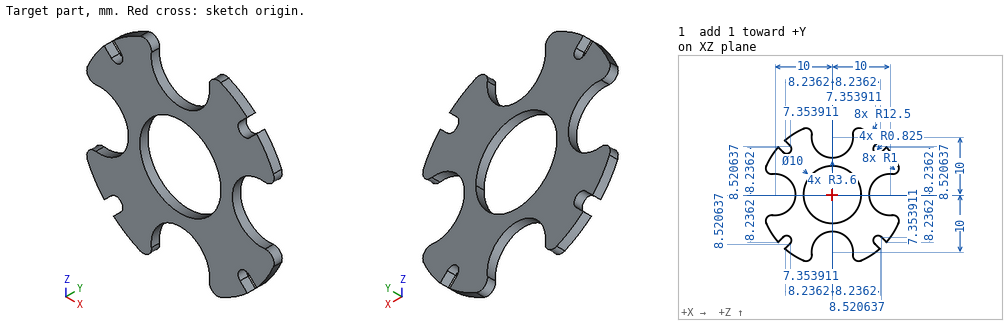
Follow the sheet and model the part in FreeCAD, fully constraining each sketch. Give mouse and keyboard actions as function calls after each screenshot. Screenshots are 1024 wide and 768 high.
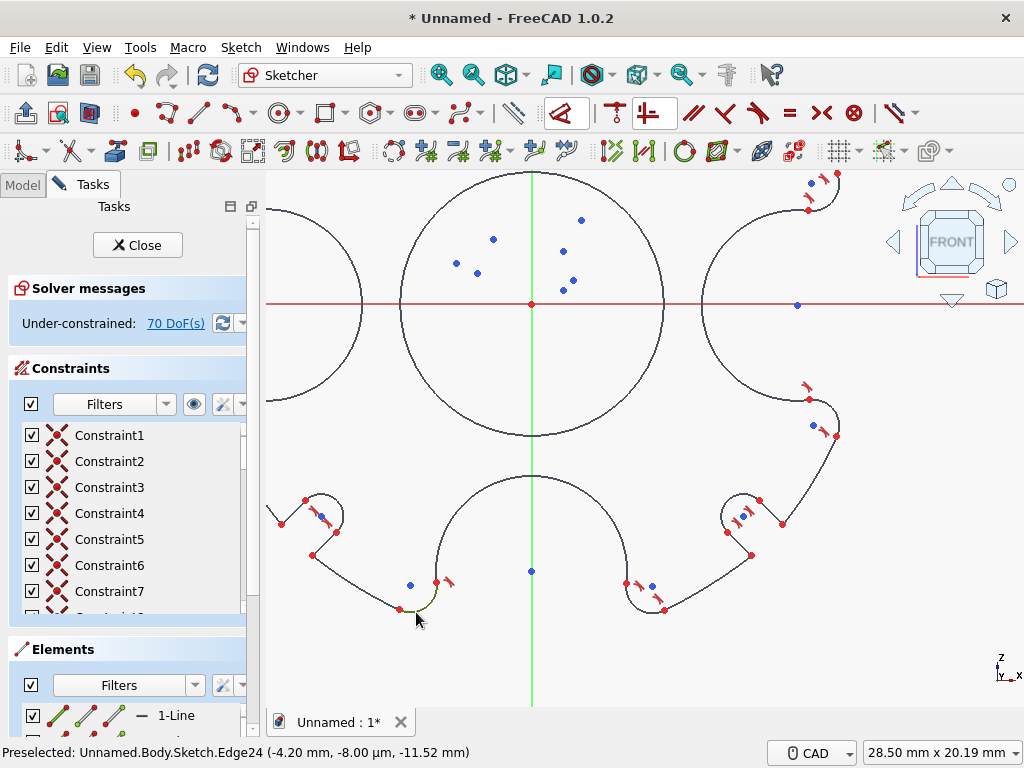
click(337, 574)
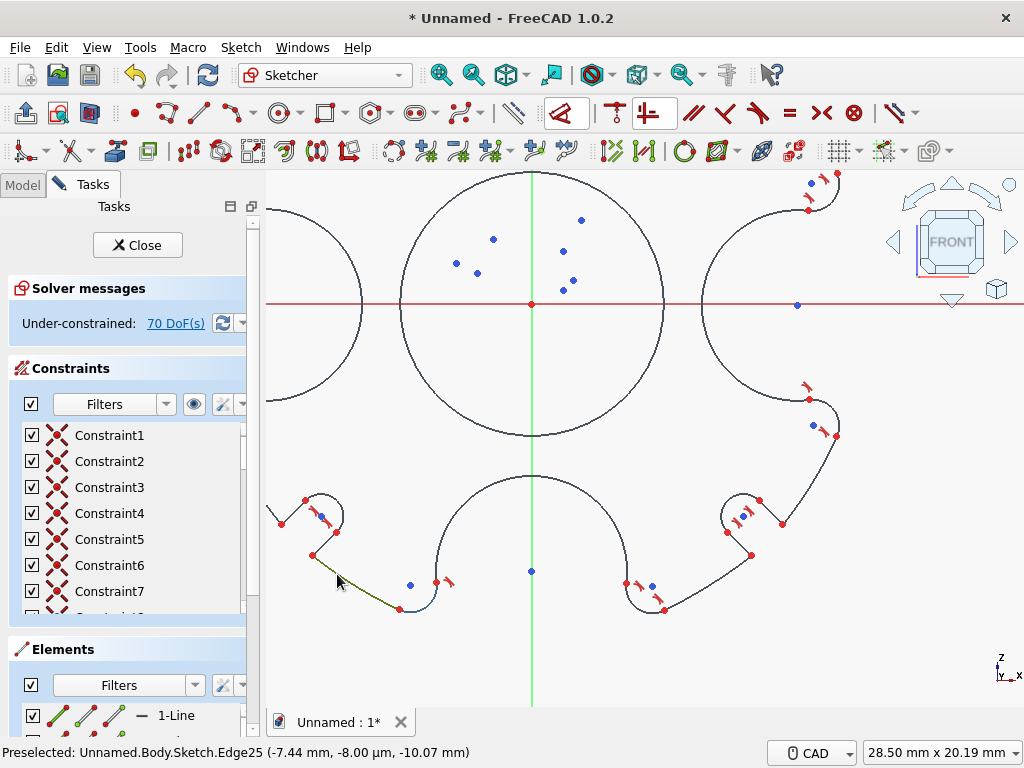
click(758, 114)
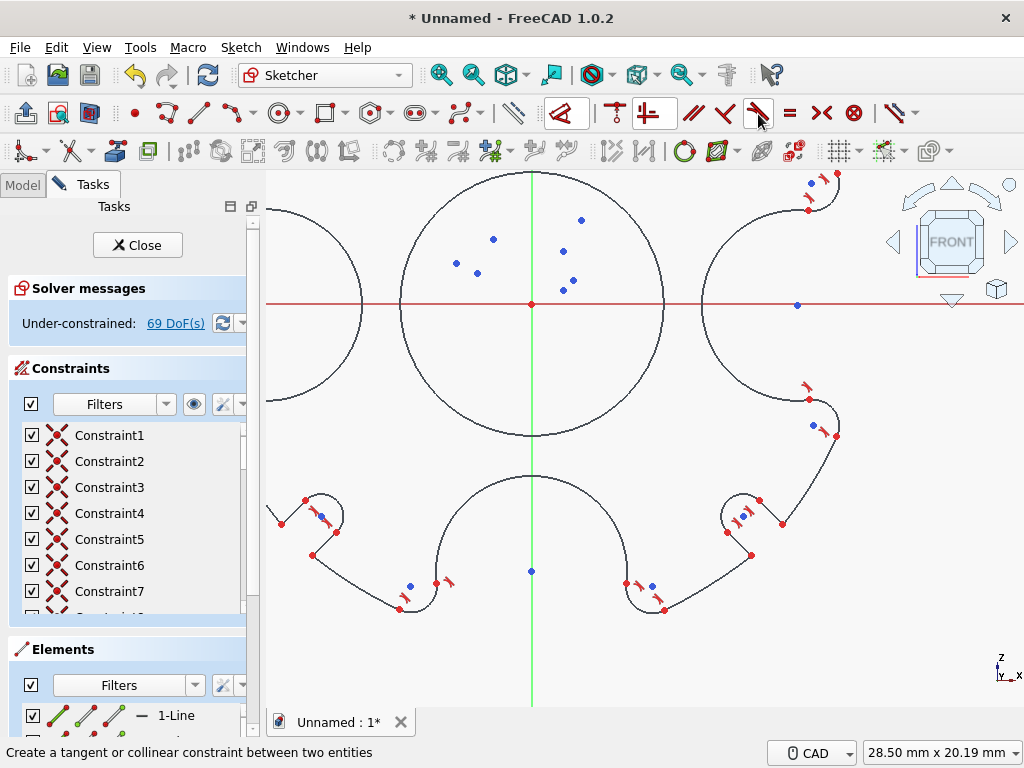
scroll(631, 602, down, 3)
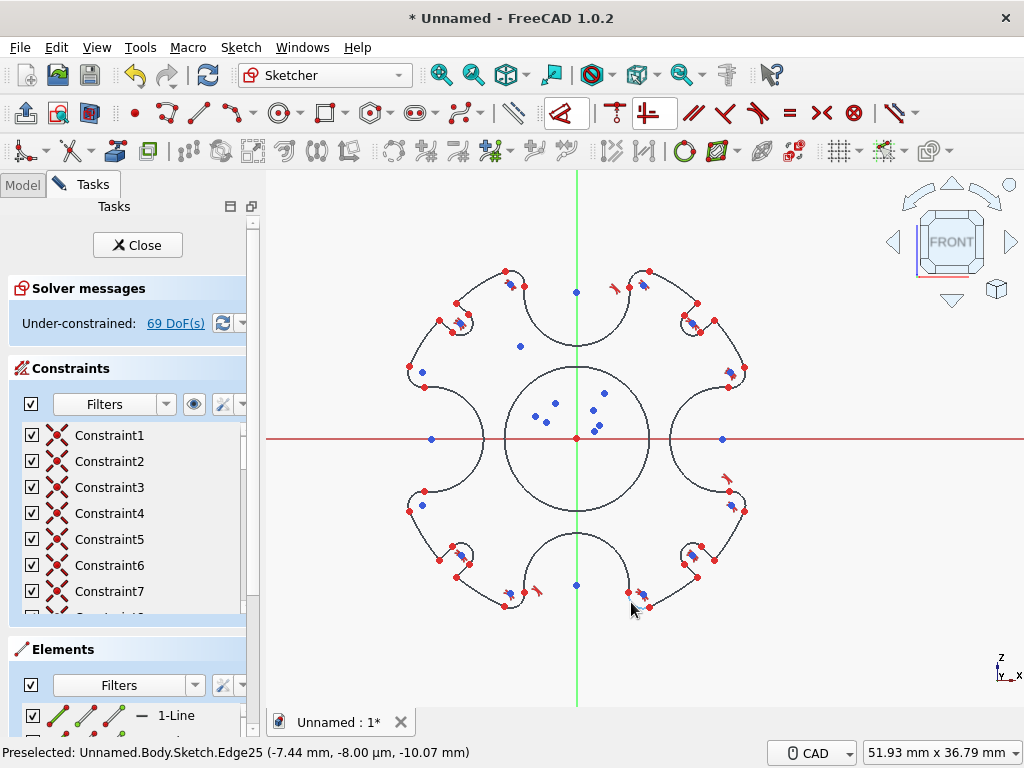
click(417, 527)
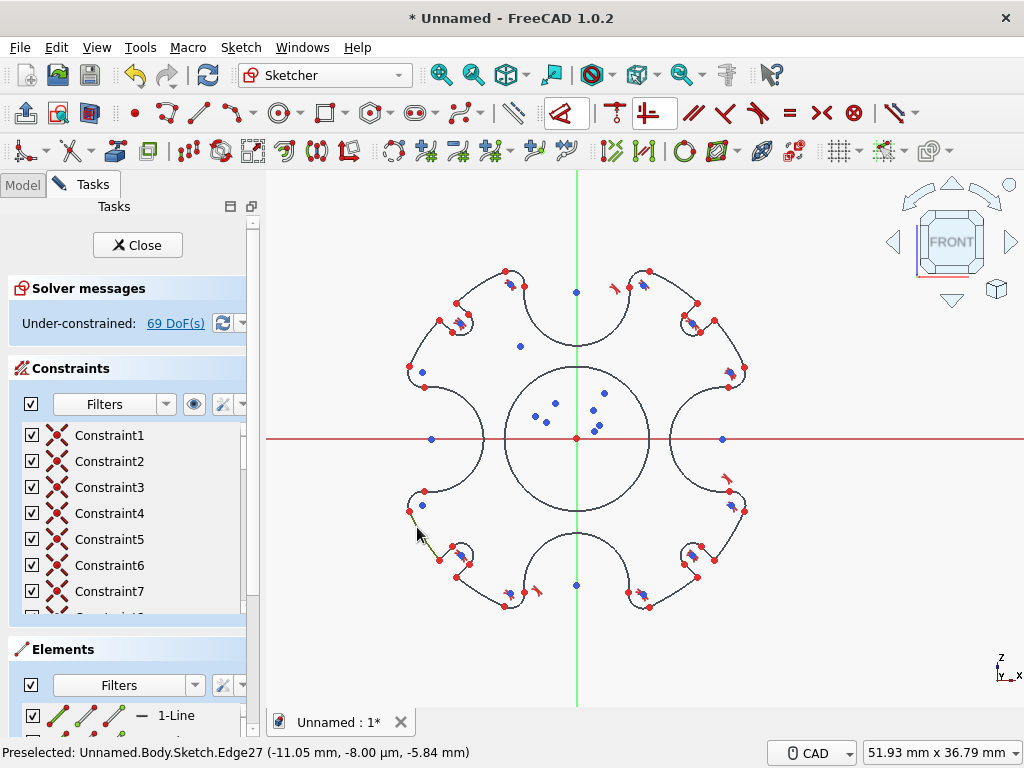
scroll(416, 493, up, 3)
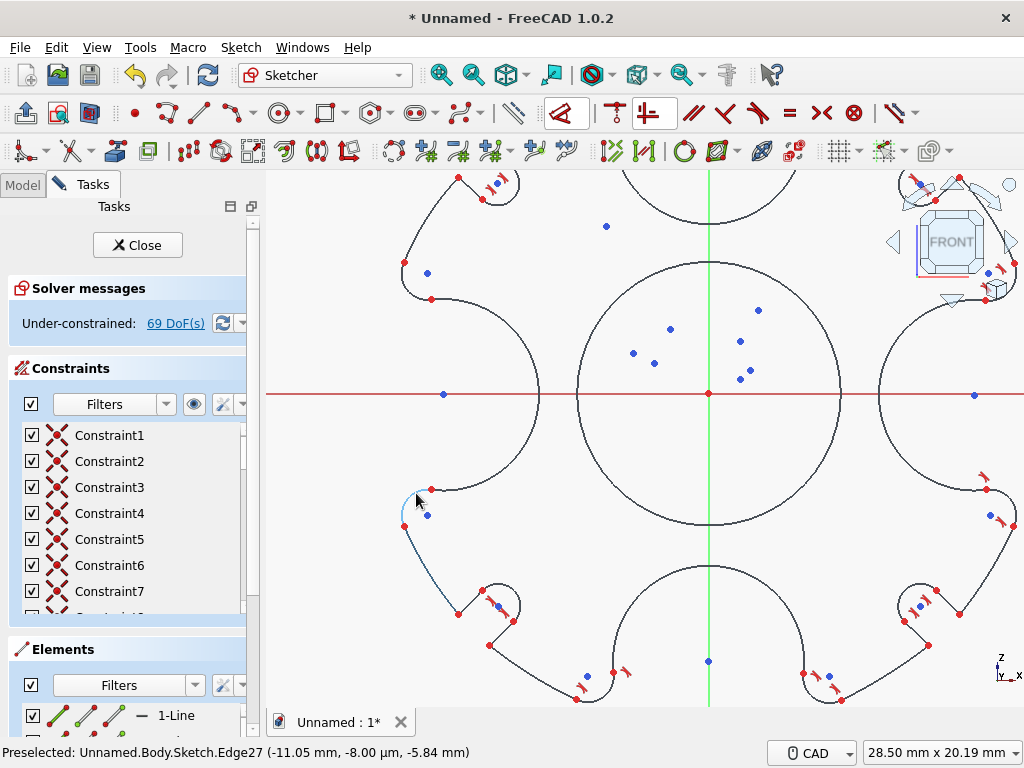
click(416, 493)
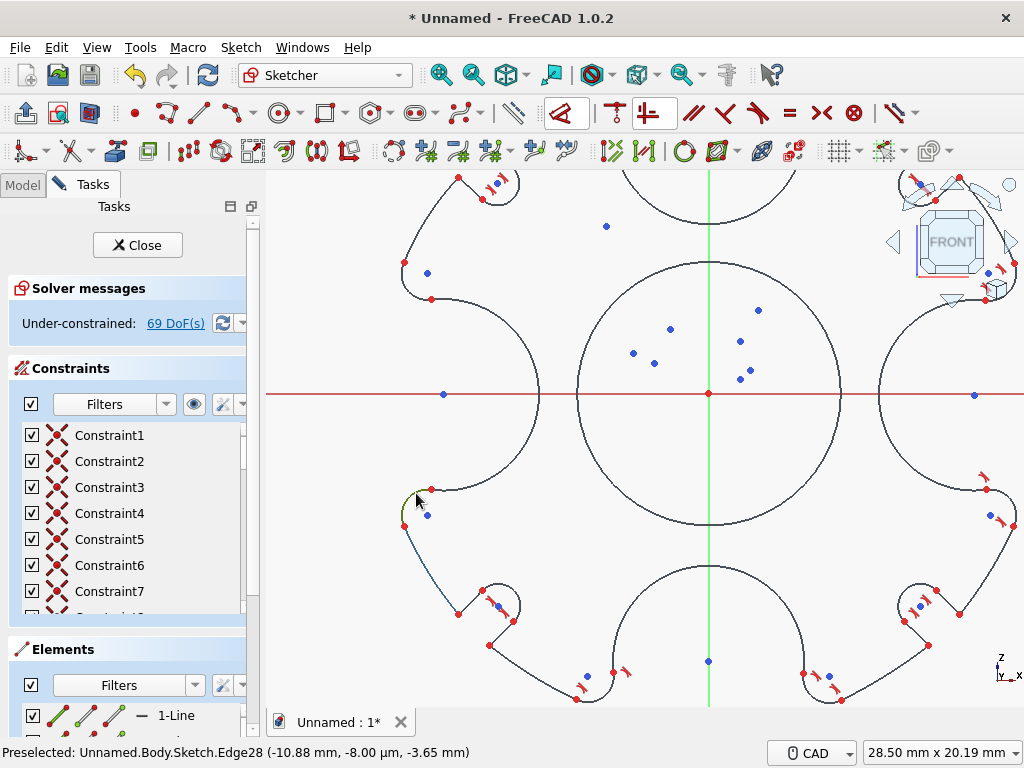
key(t)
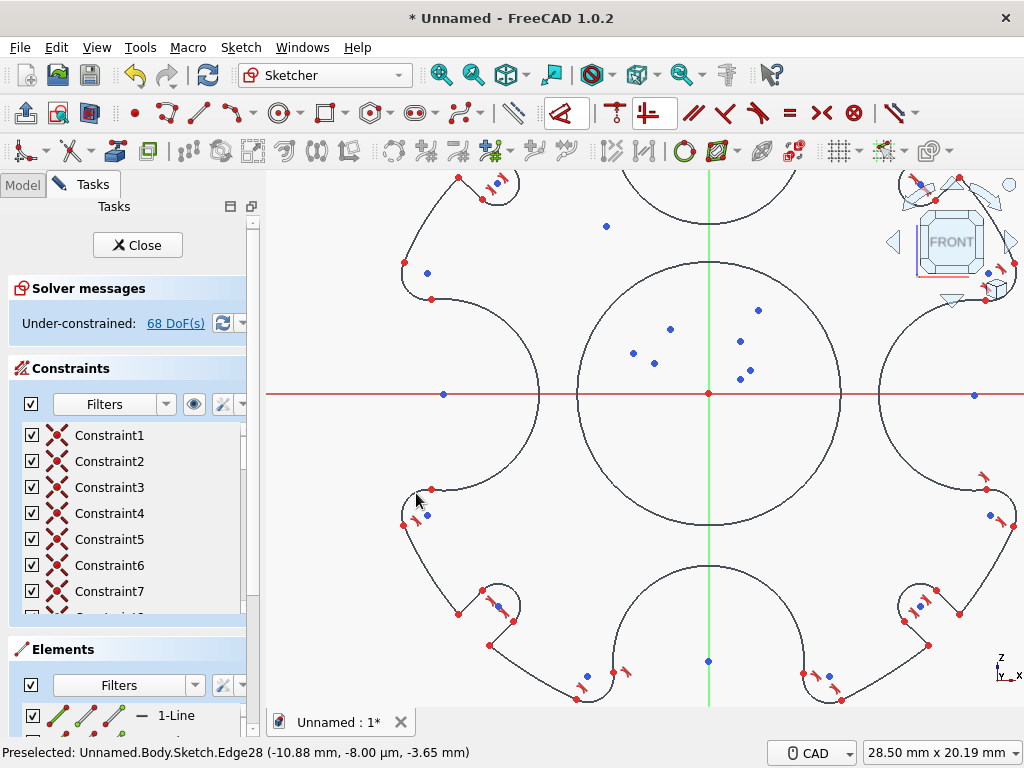
click(416, 492)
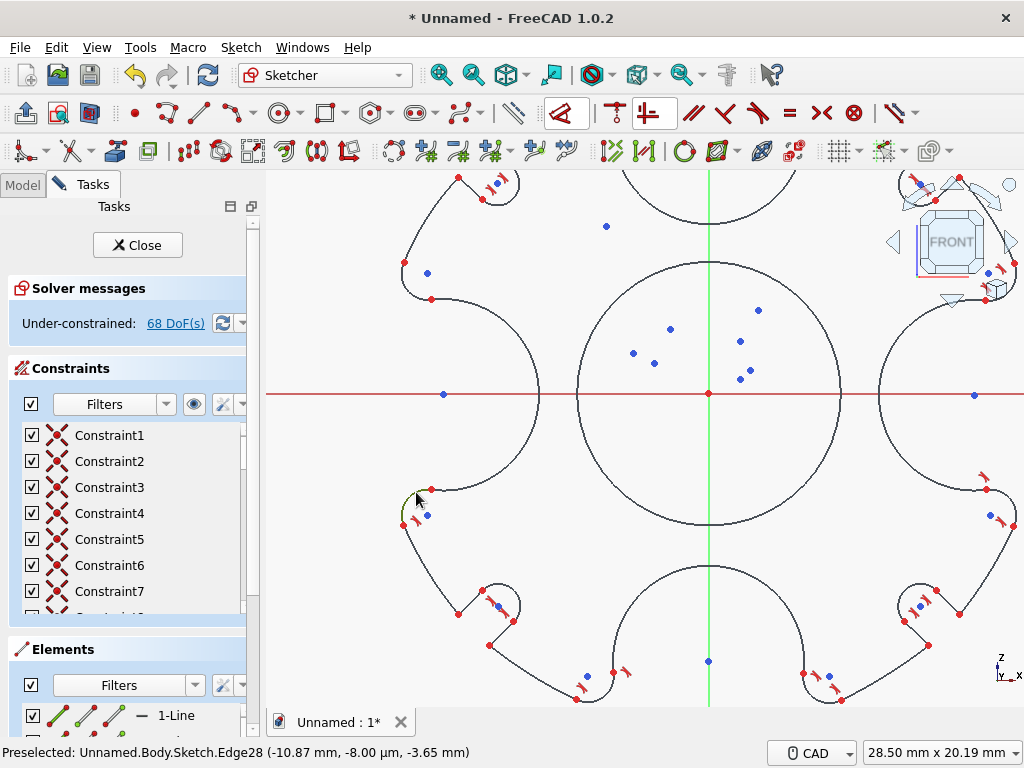
click(518, 455)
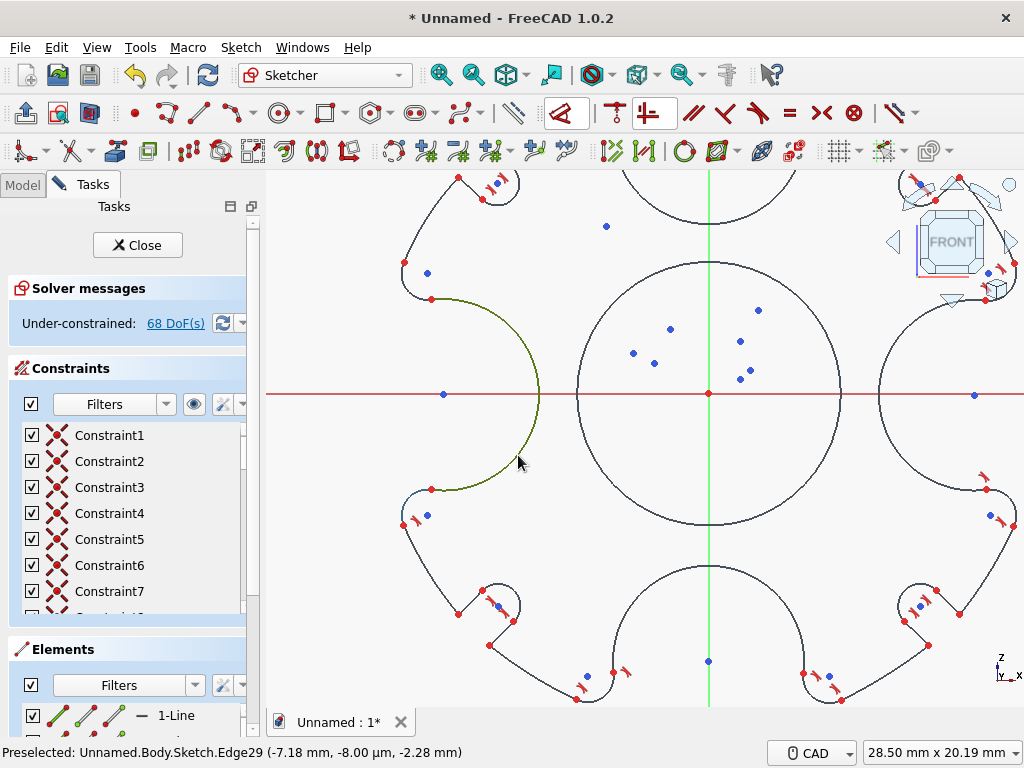
key(t)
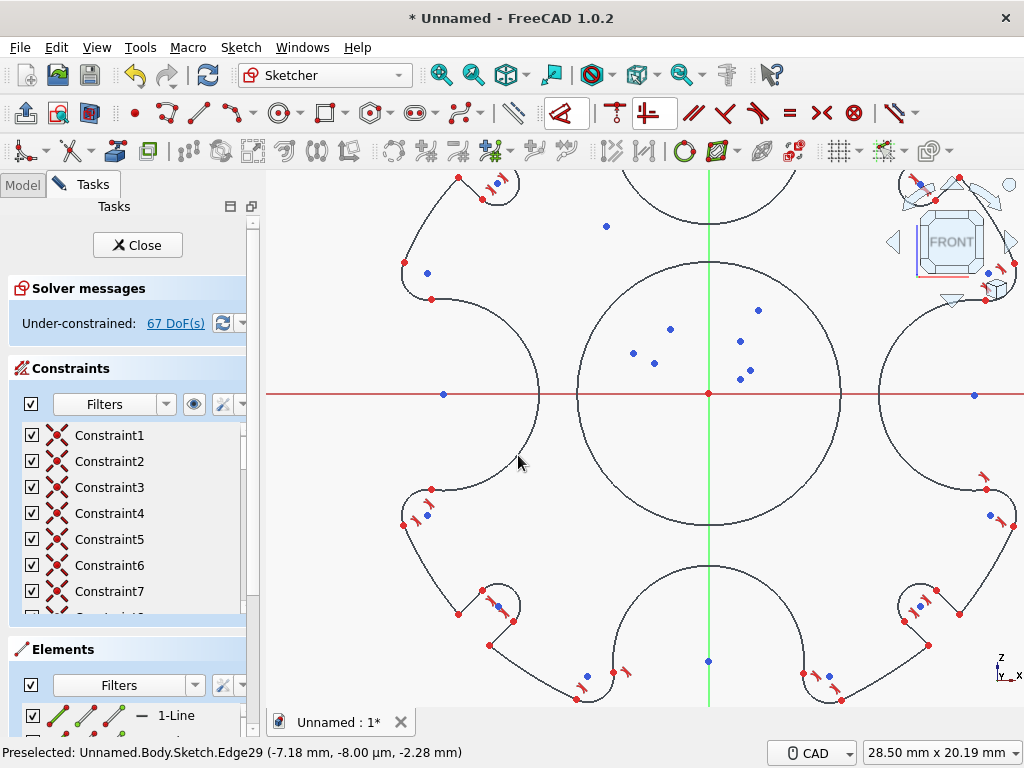
click(518, 455)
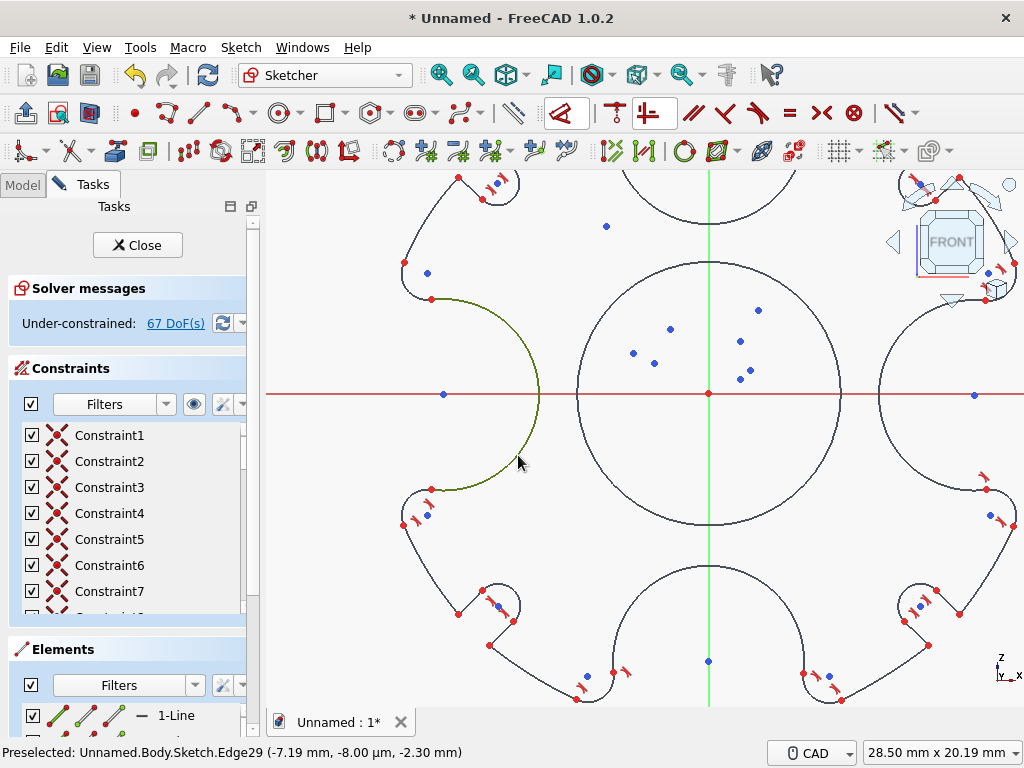
click(402, 279)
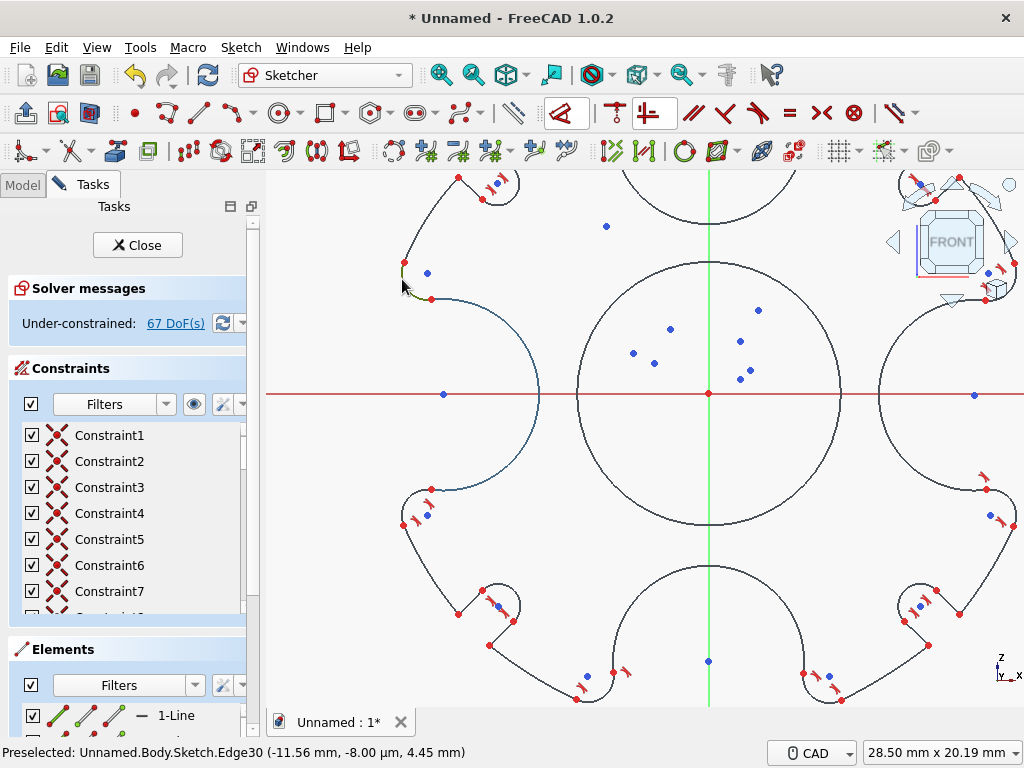
key(t)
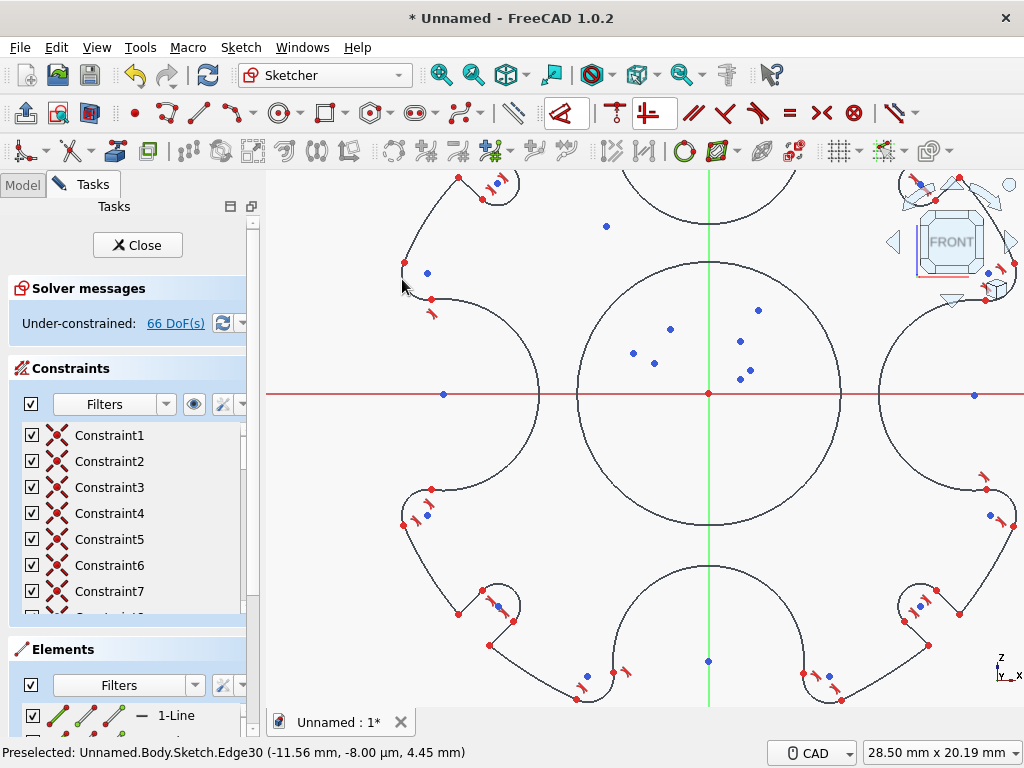
click(402, 279)